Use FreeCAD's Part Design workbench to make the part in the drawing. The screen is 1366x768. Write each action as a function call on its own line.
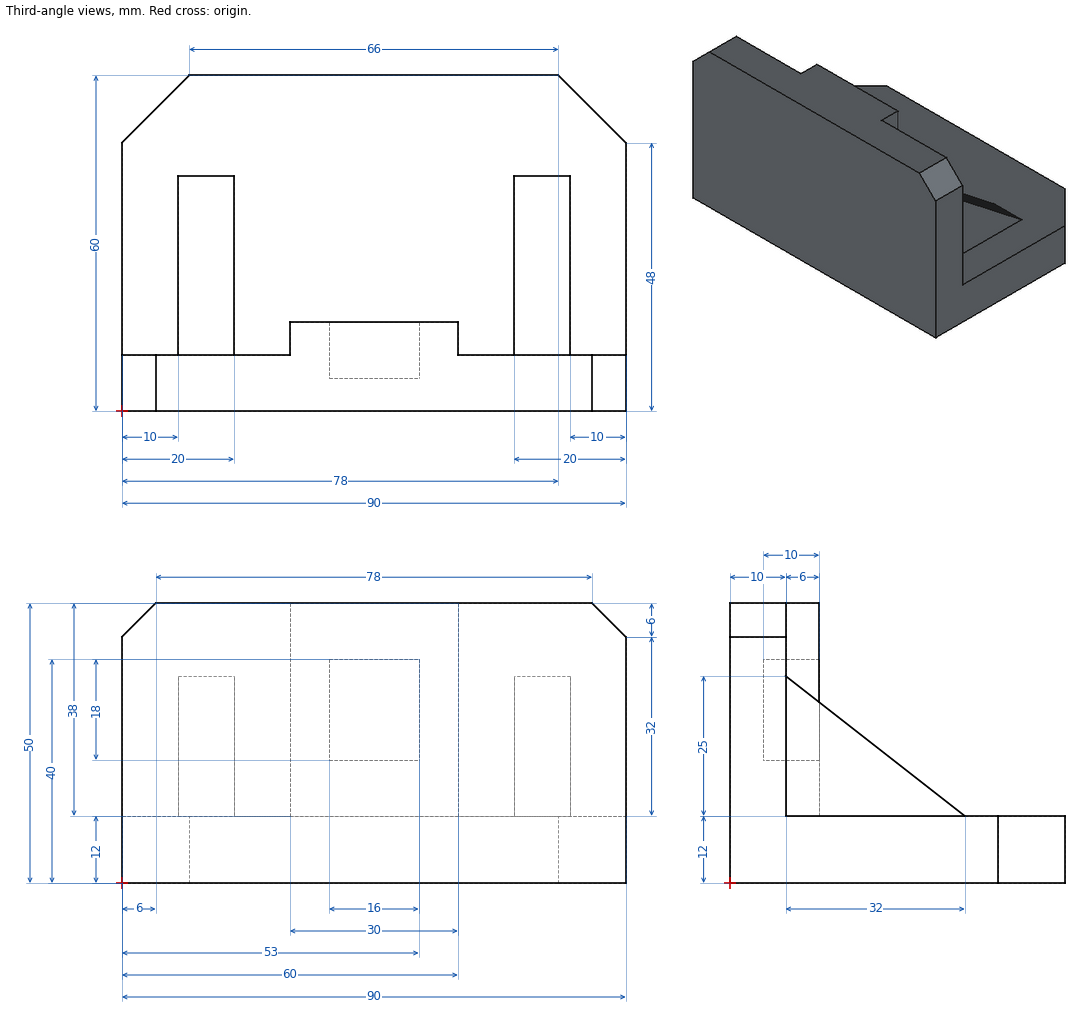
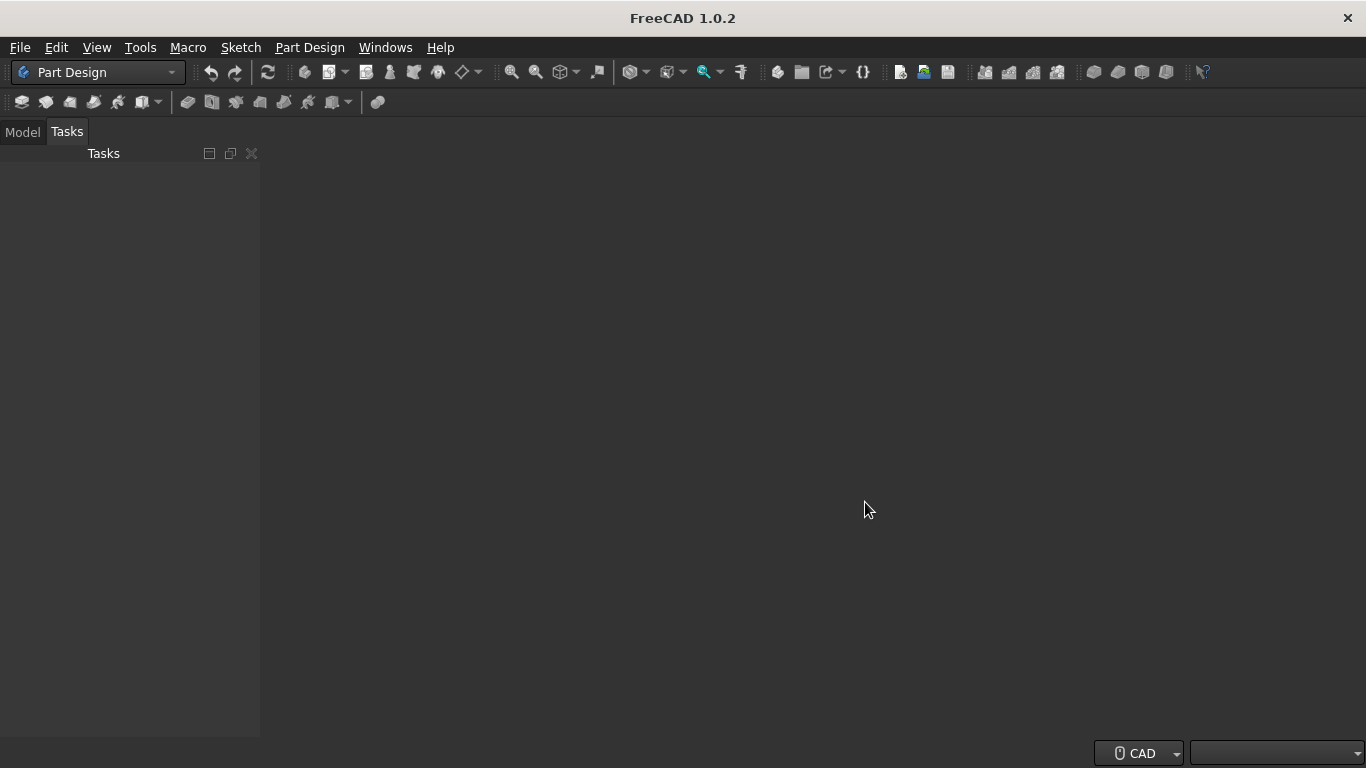
click(900, 72)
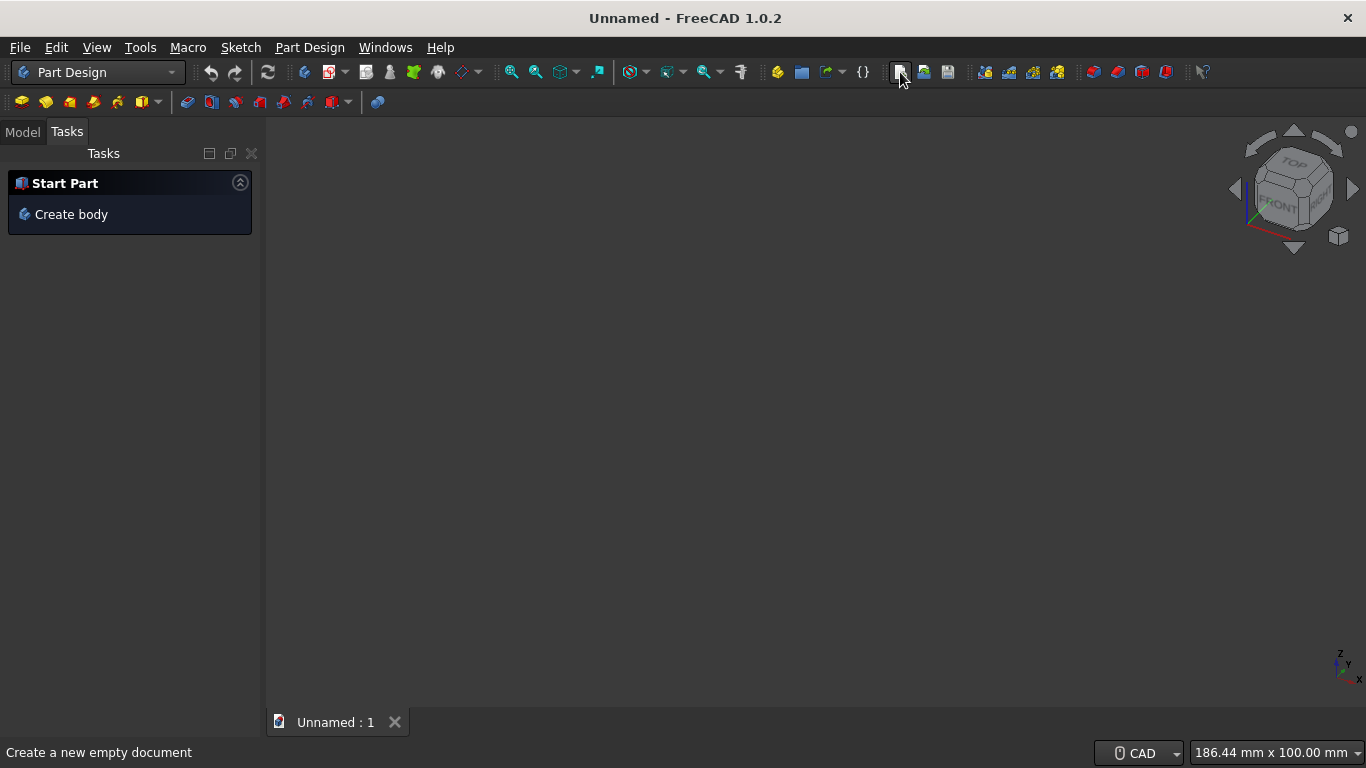
click(330, 72)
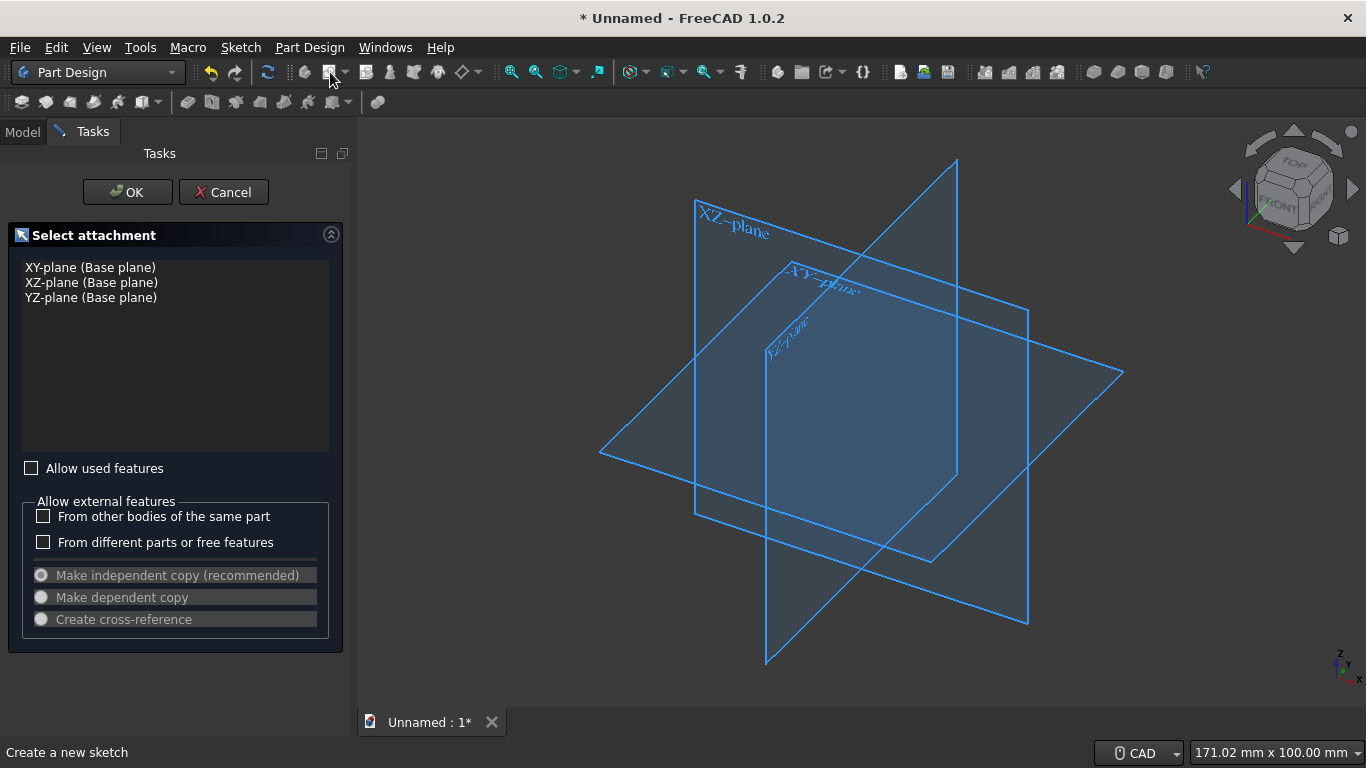
click(82, 268)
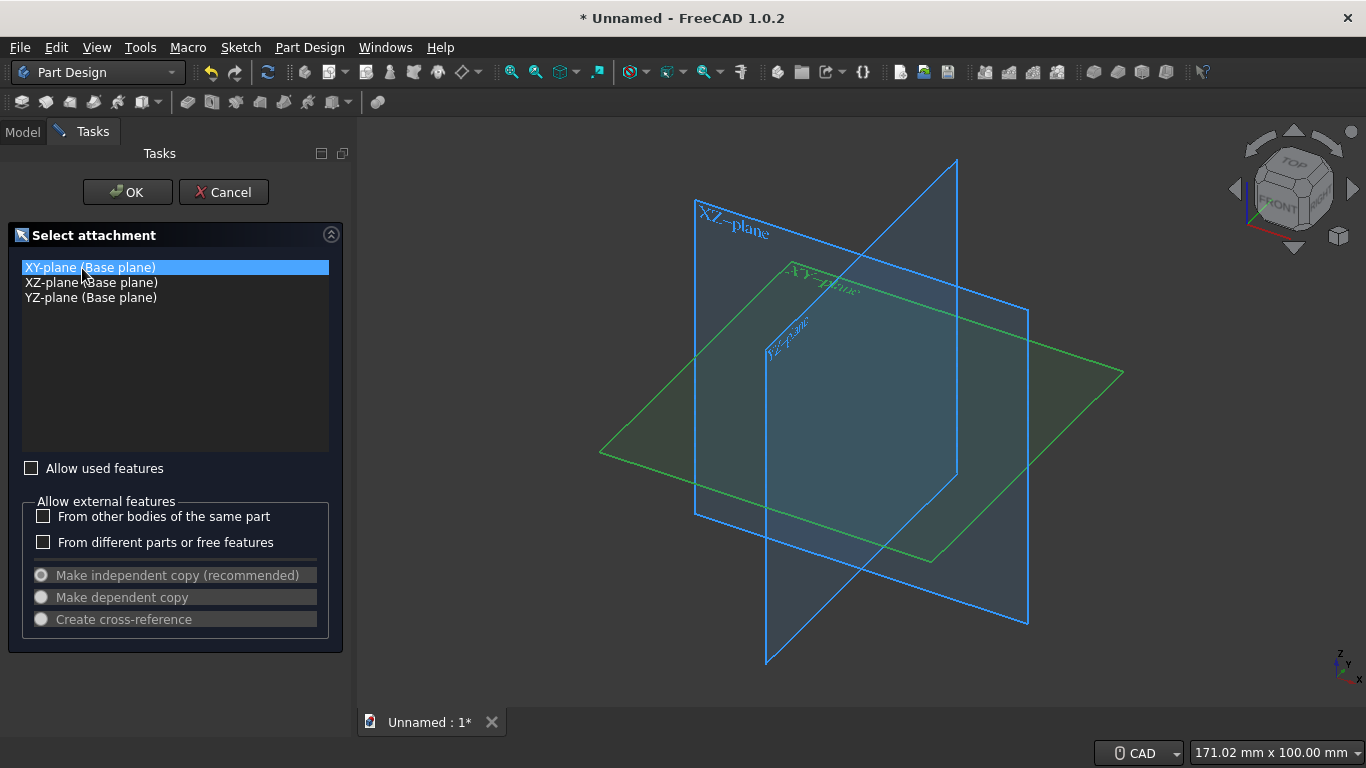
click(128, 192)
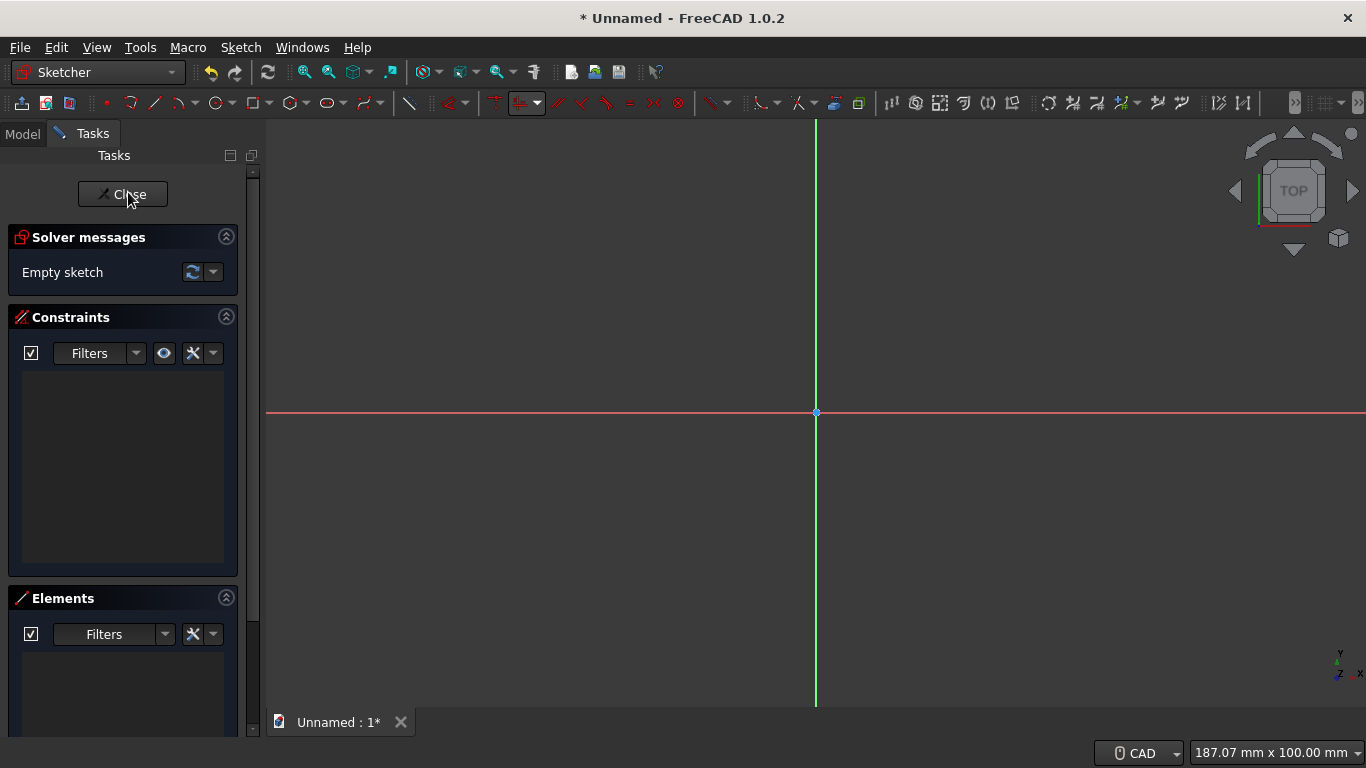
scroll(294, 679, down, 1)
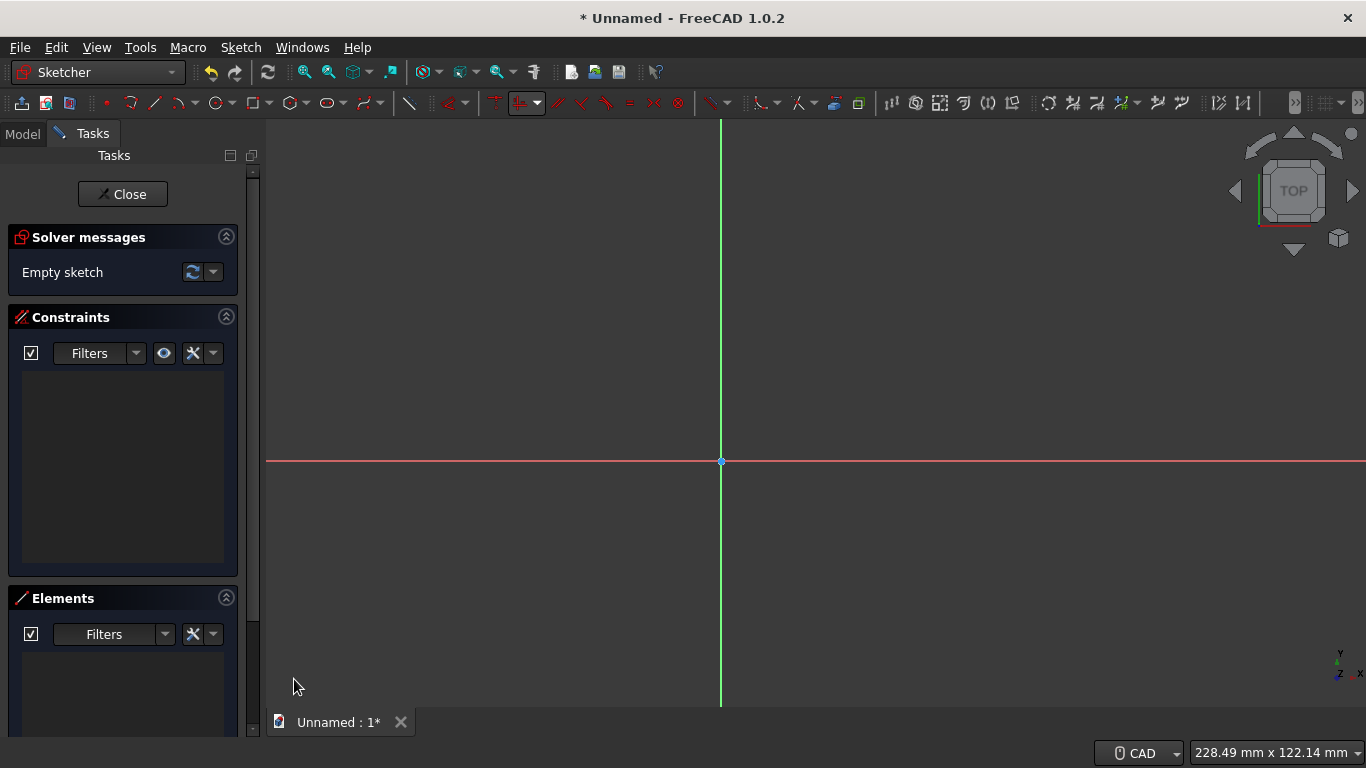
click(132, 104)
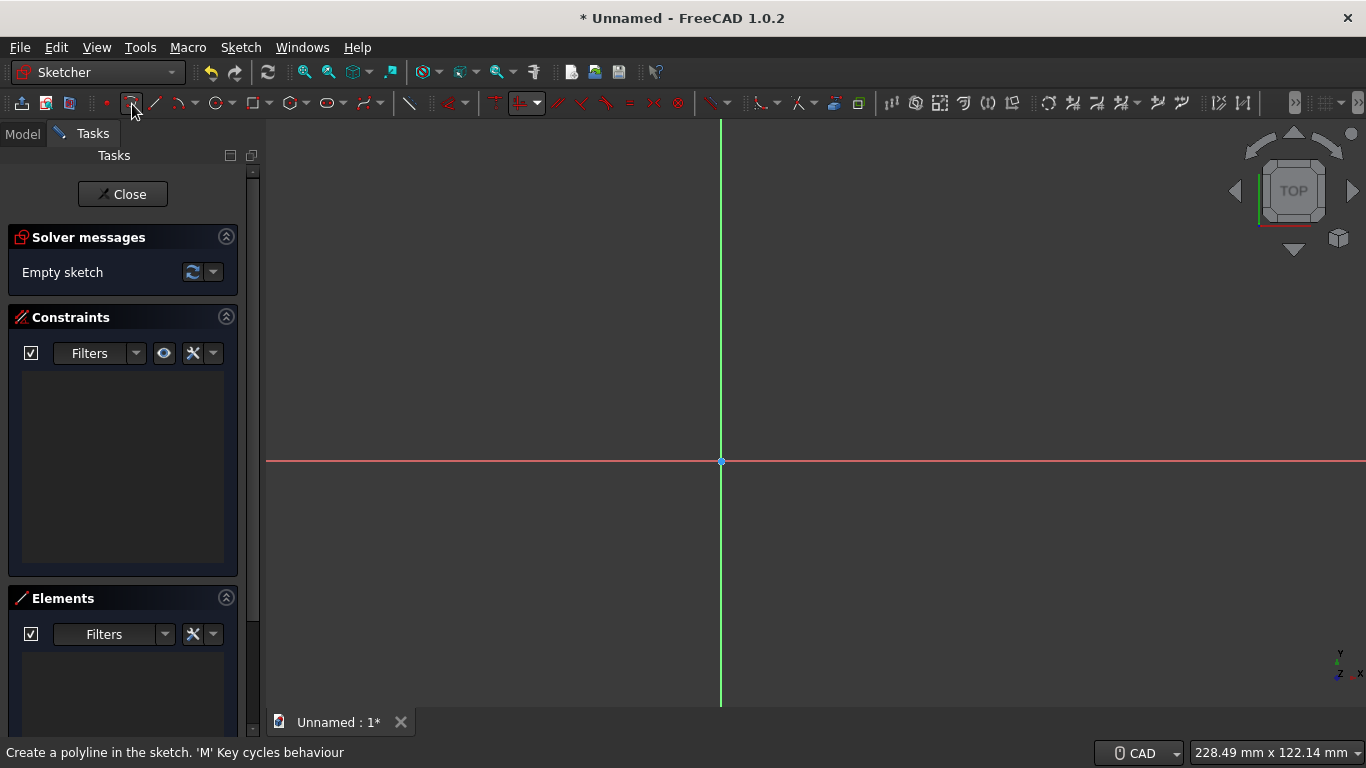
click(721, 461)
click(1155, 452)
click(1155, 230)
click(1097, 173)
click(779, 173)
click(730, 230)
click(721, 461)
key(Escape)
key(Escape)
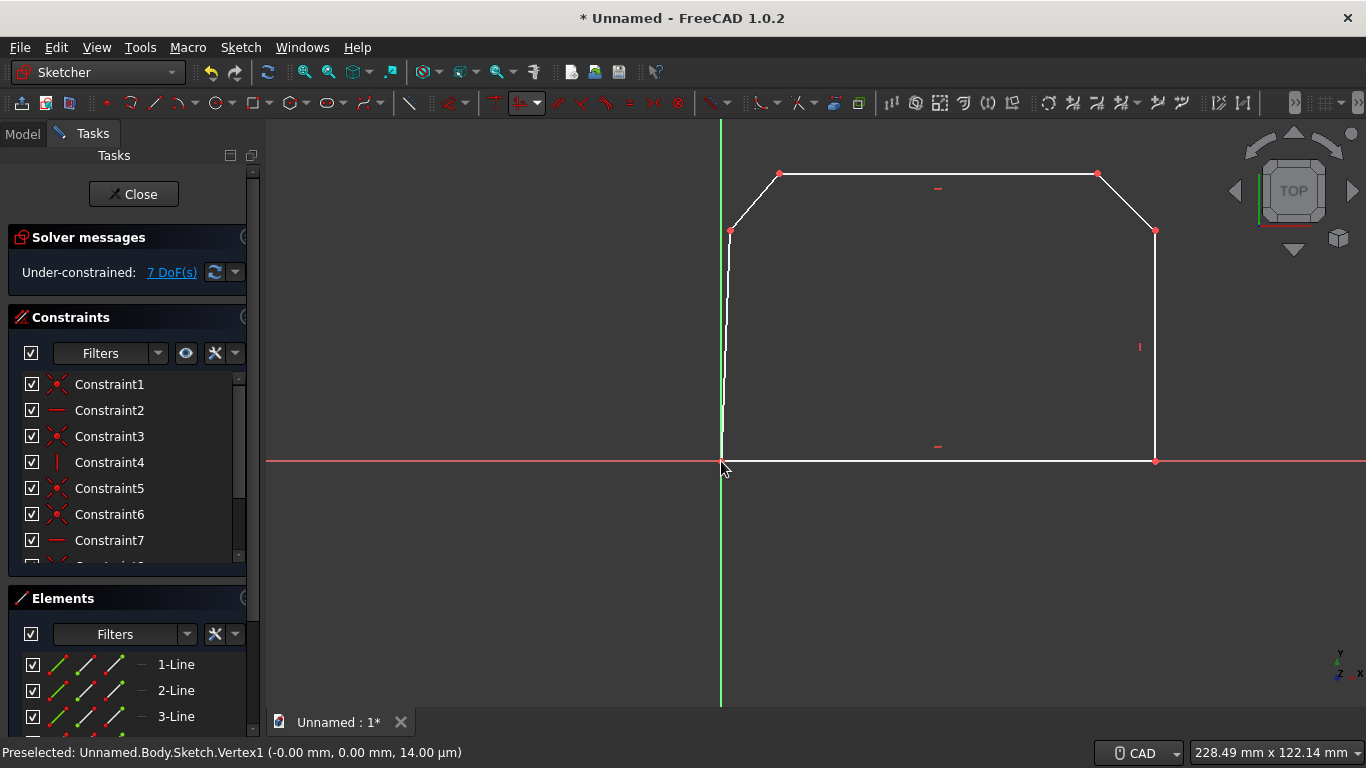
click(724, 392)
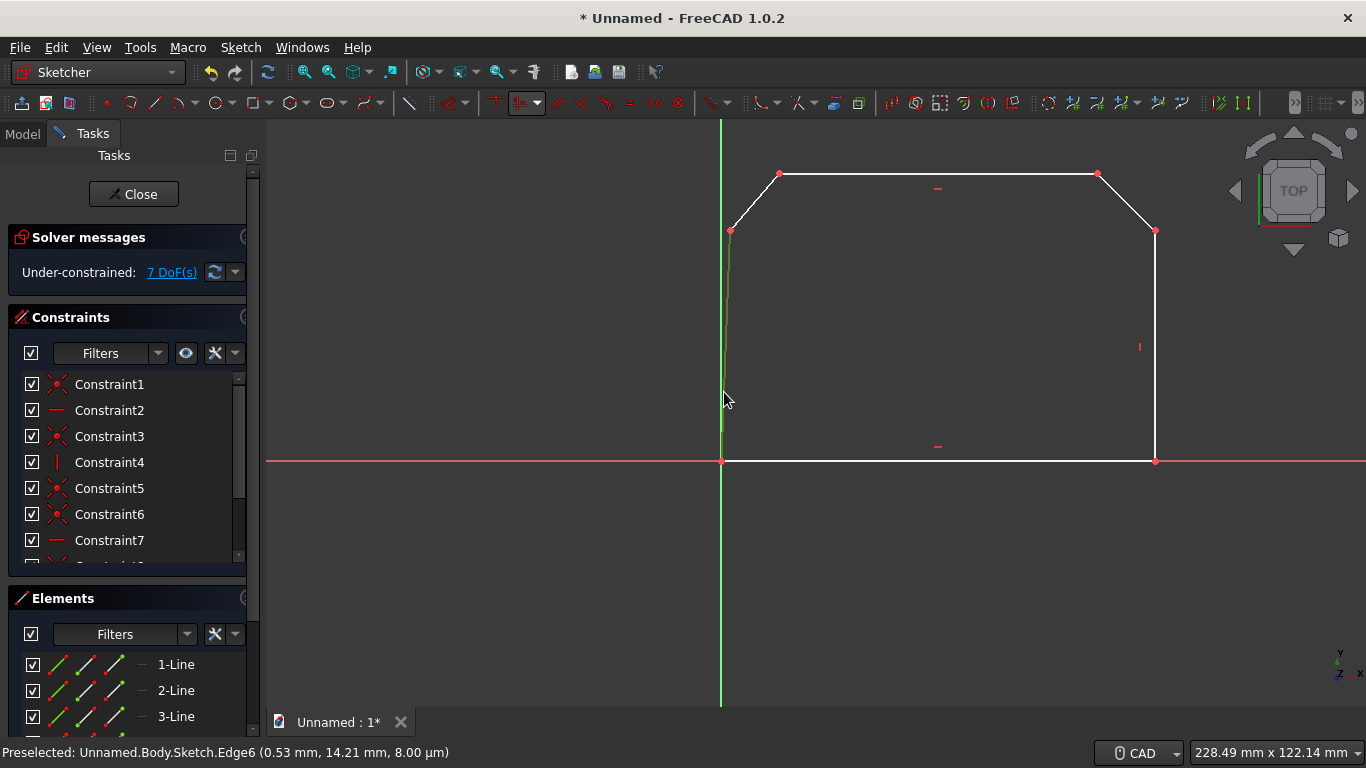
key(v)